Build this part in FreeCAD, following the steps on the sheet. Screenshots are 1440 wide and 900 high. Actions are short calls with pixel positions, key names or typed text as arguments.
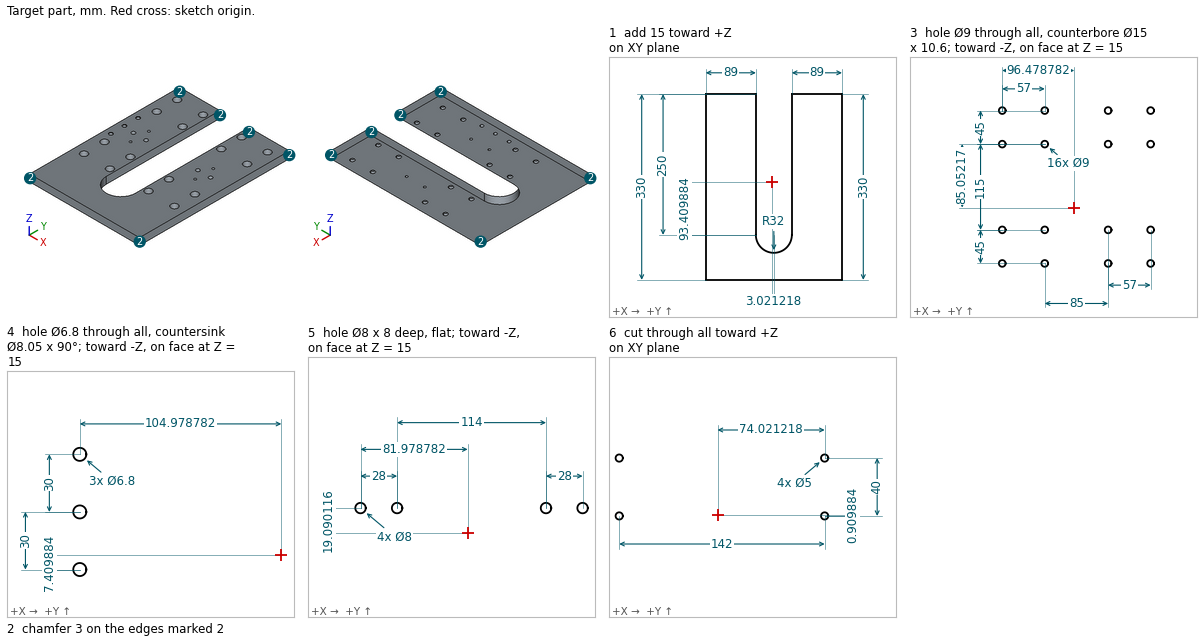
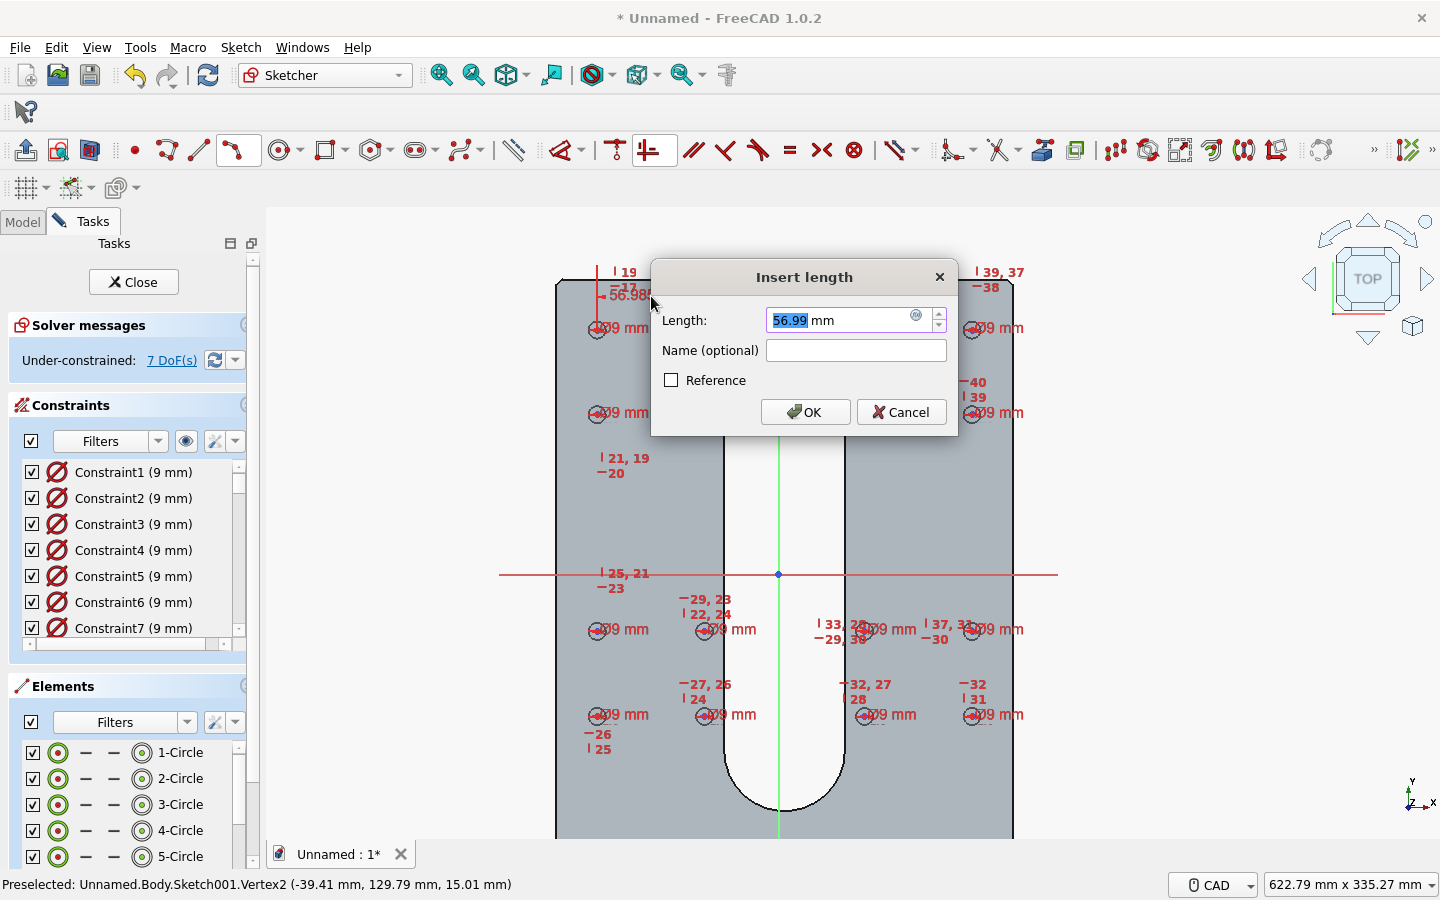
text(57)
key(Return)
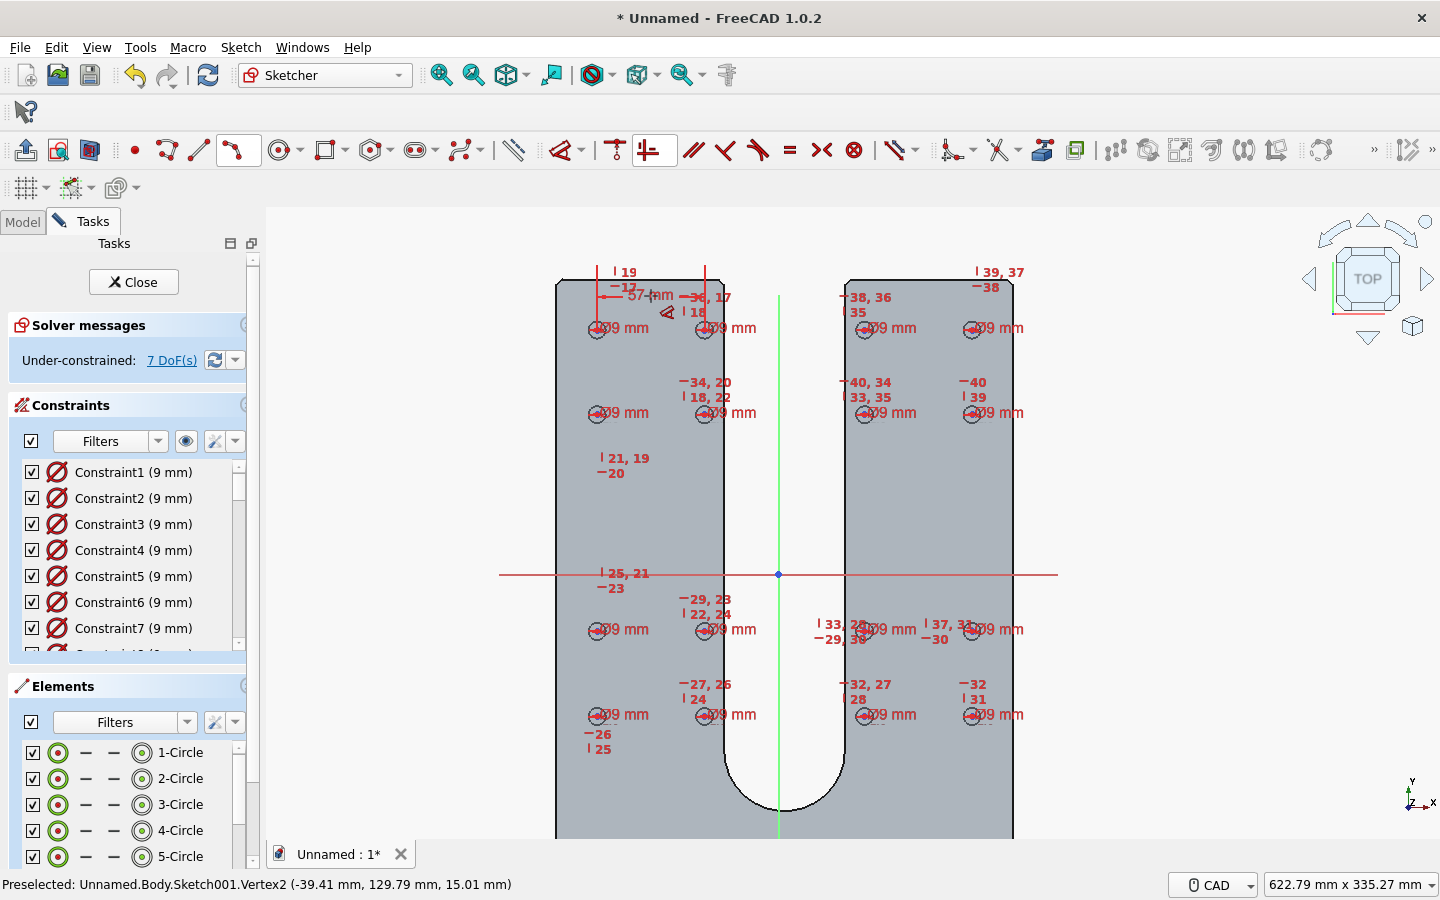
click(705, 330)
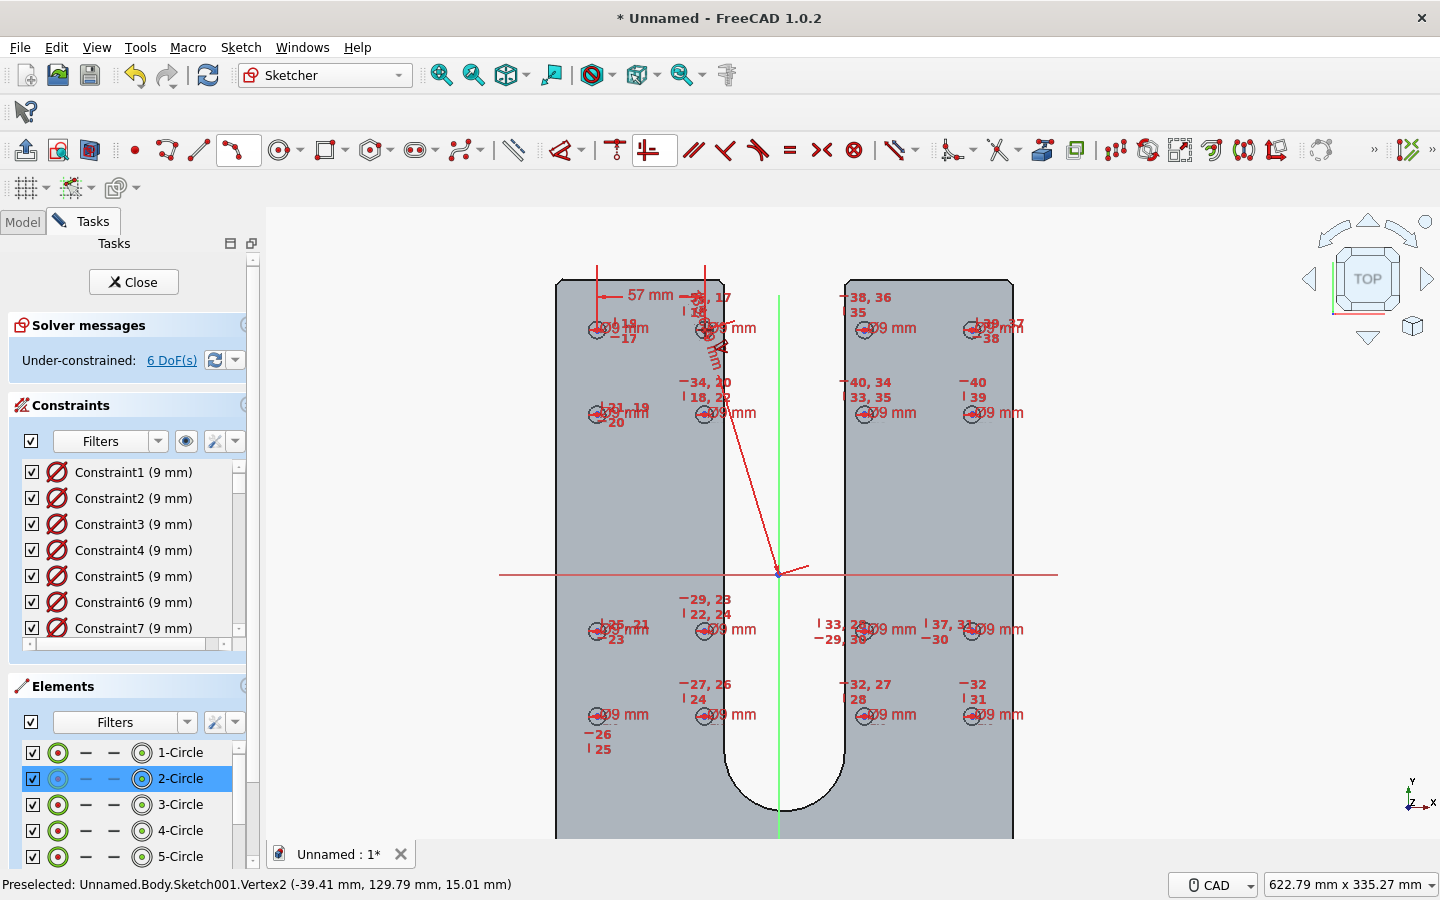
click(705, 415)
click(671, 372)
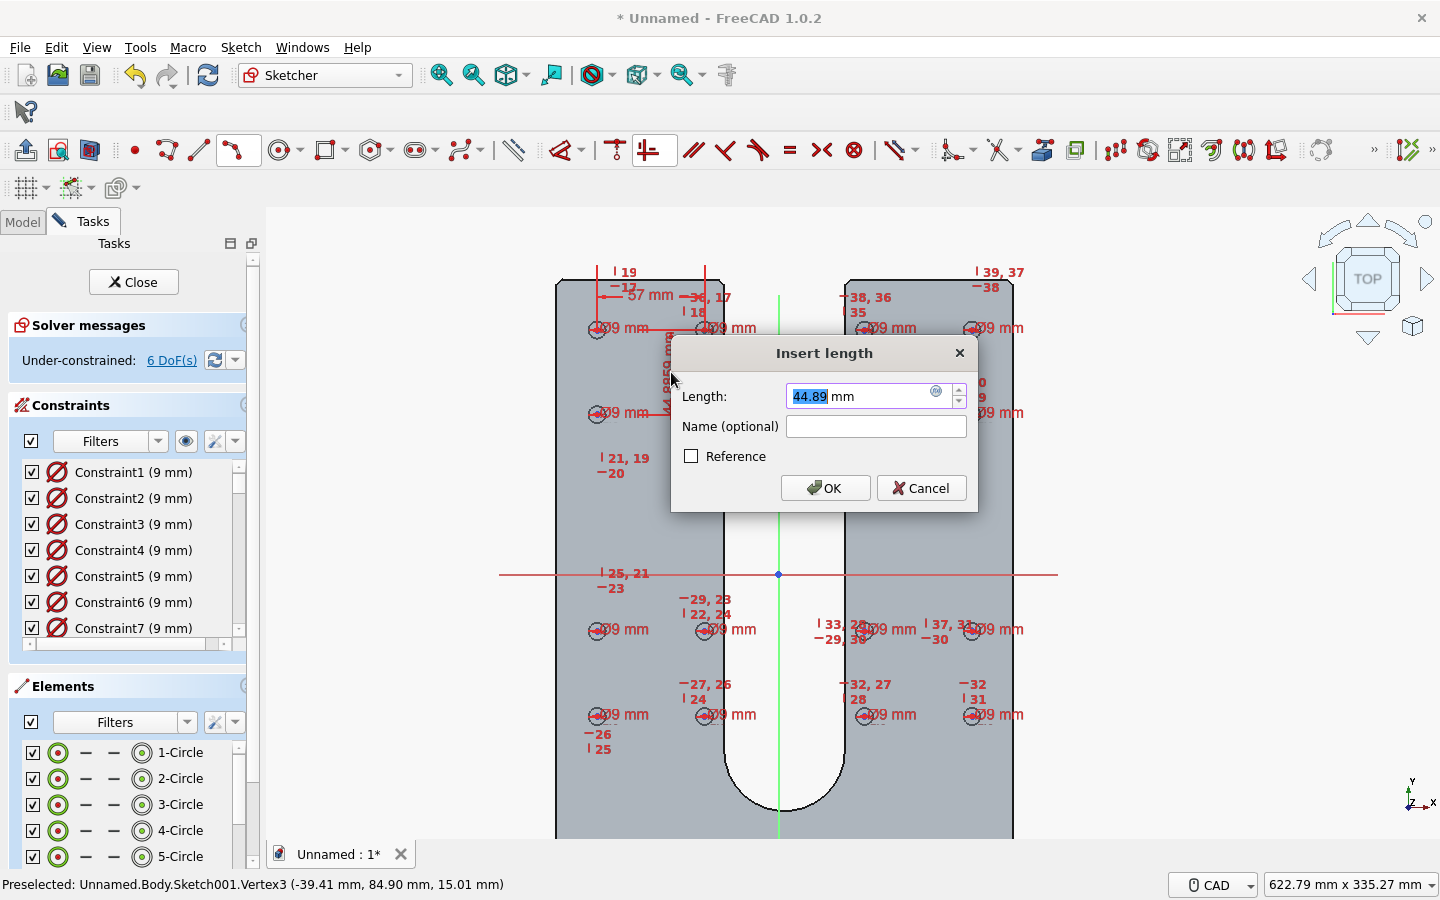
text(45)
key(Return)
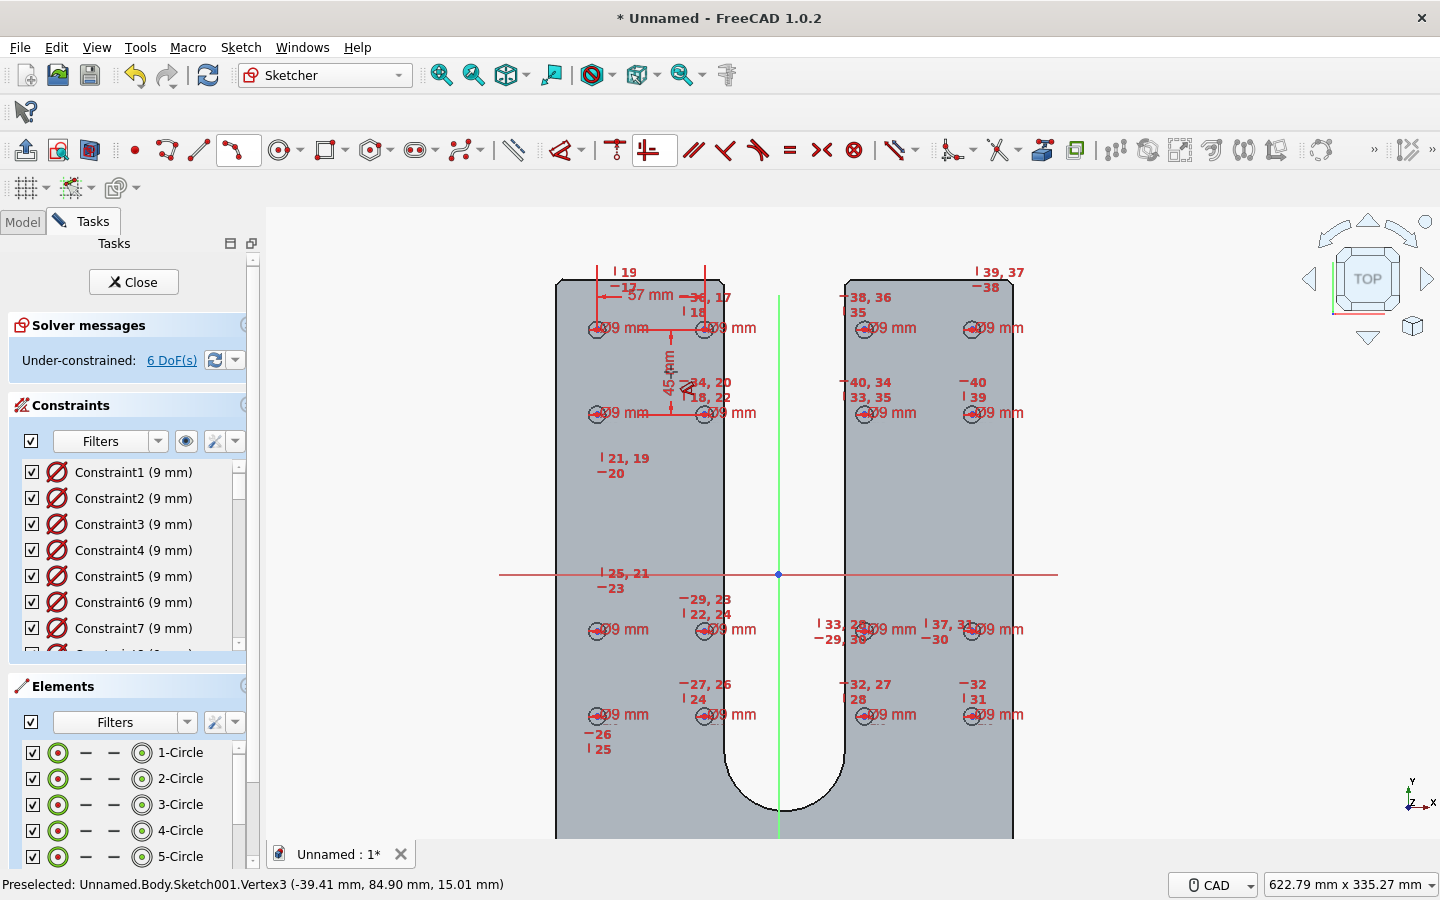
click(705, 631)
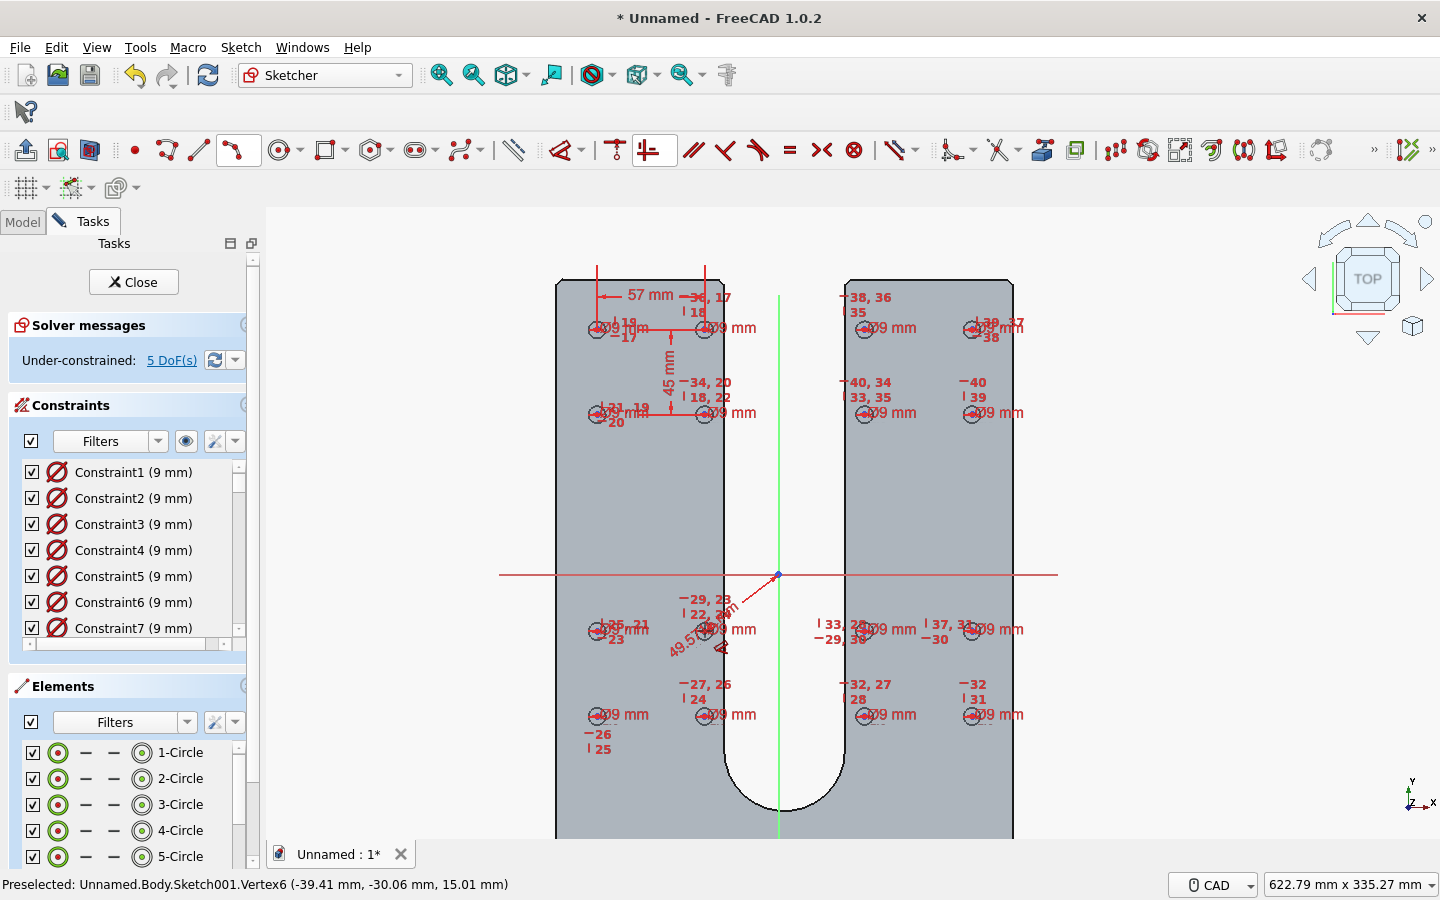
click(705, 717)
click(671, 674)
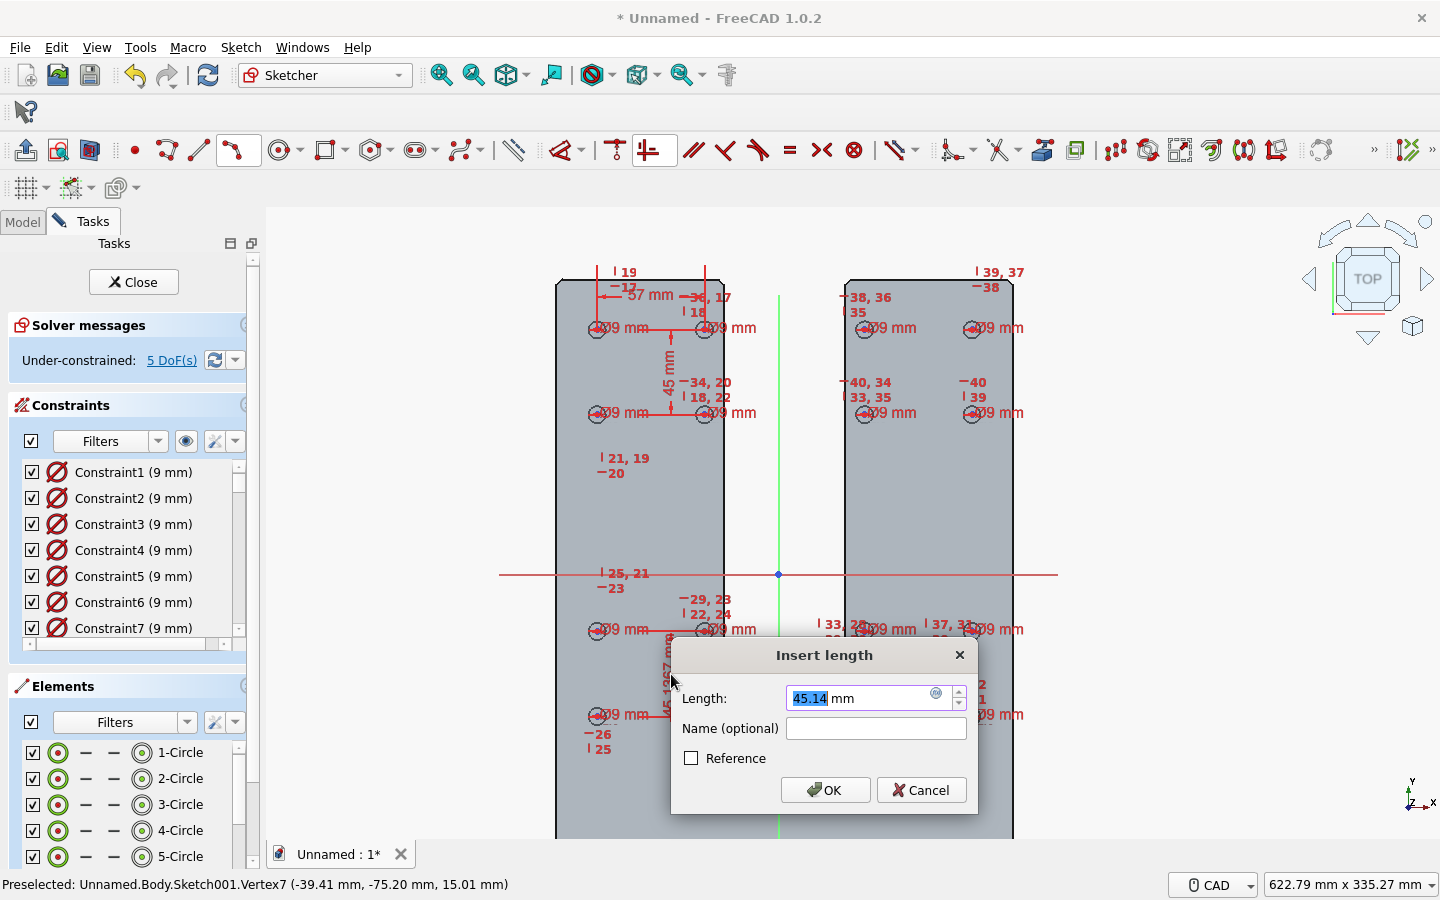
text(45)
key(Return)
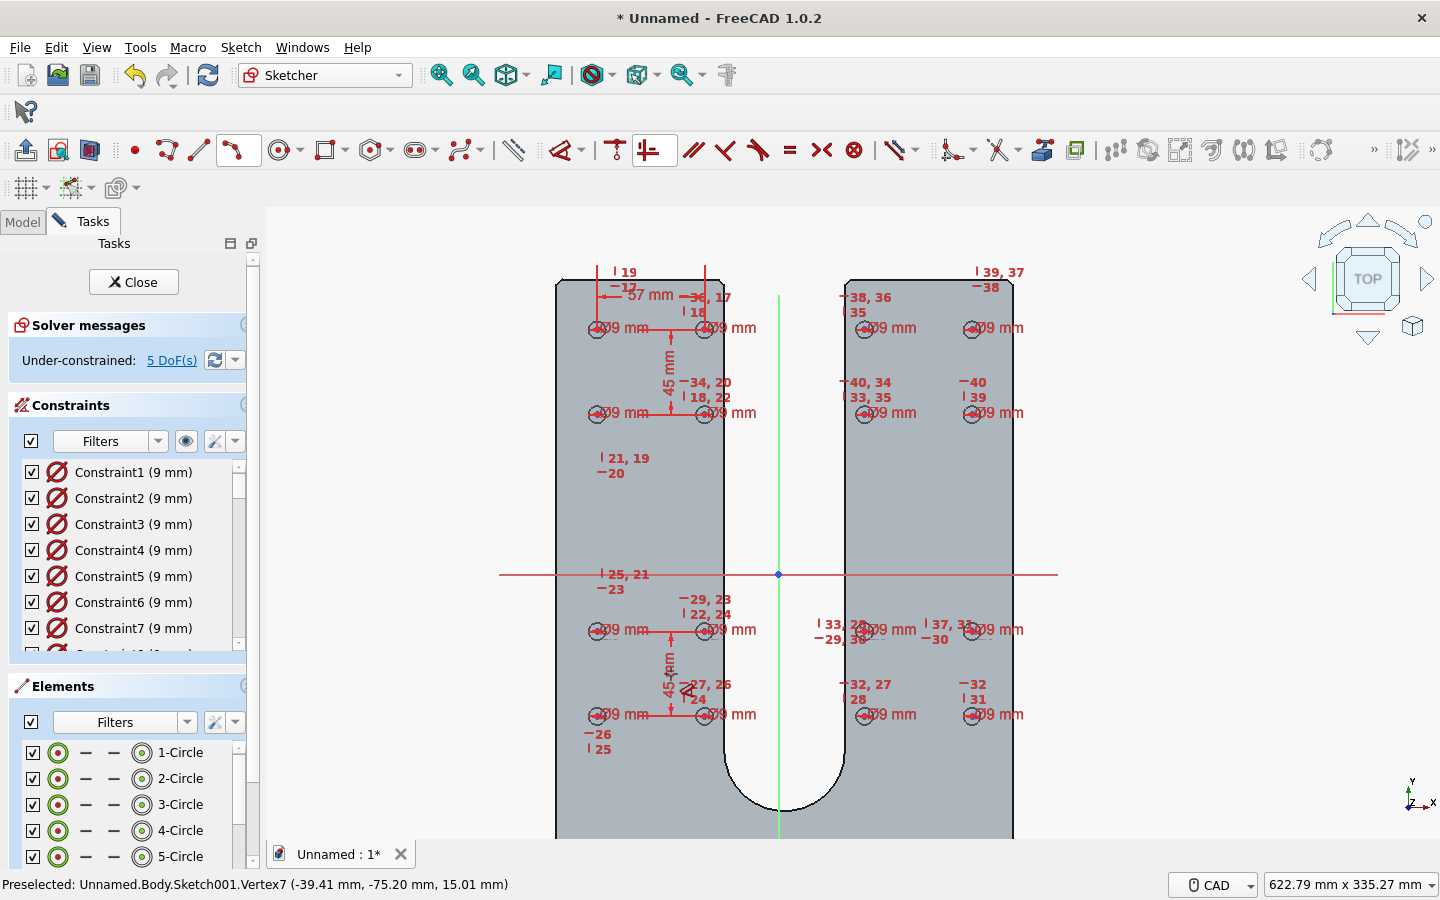
click(705, 716)